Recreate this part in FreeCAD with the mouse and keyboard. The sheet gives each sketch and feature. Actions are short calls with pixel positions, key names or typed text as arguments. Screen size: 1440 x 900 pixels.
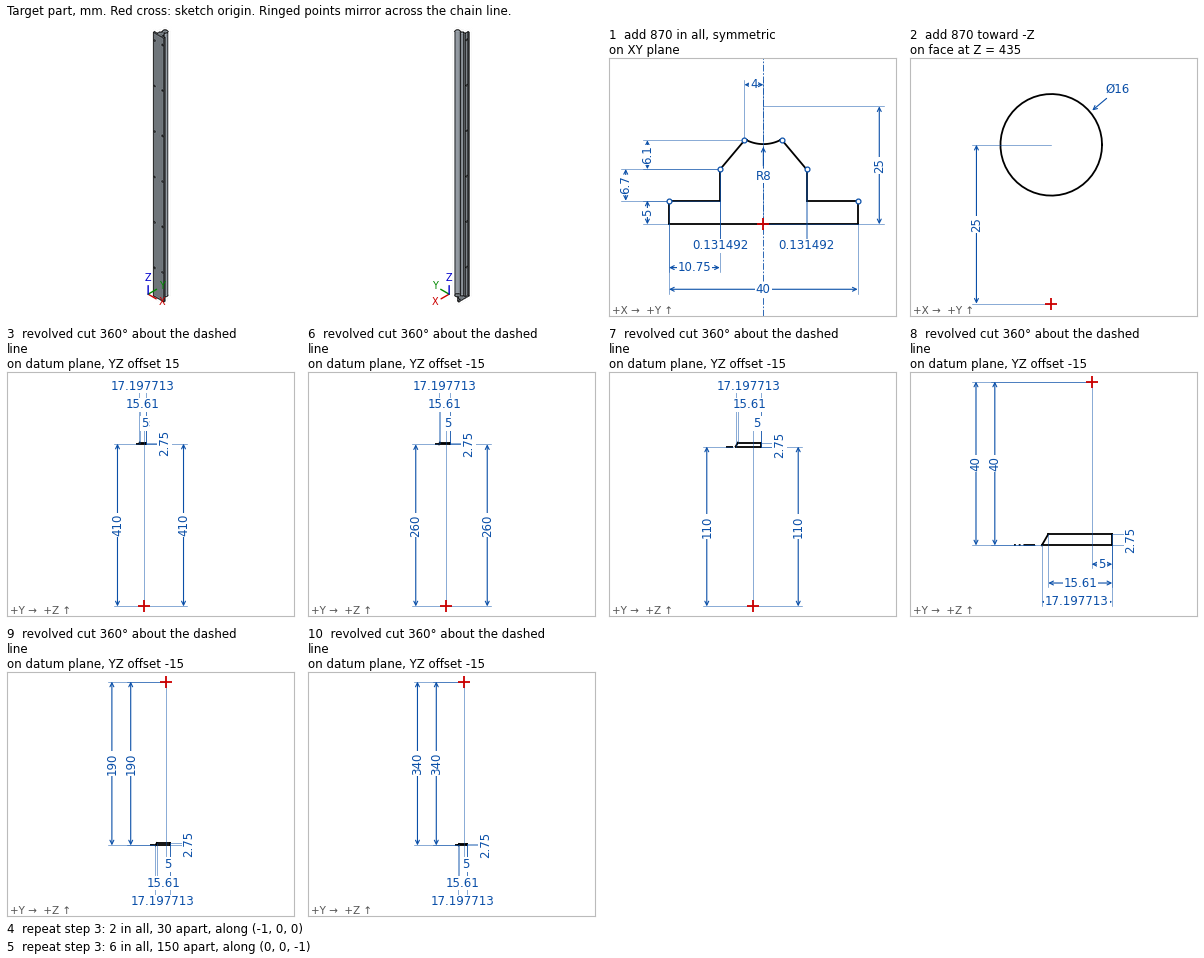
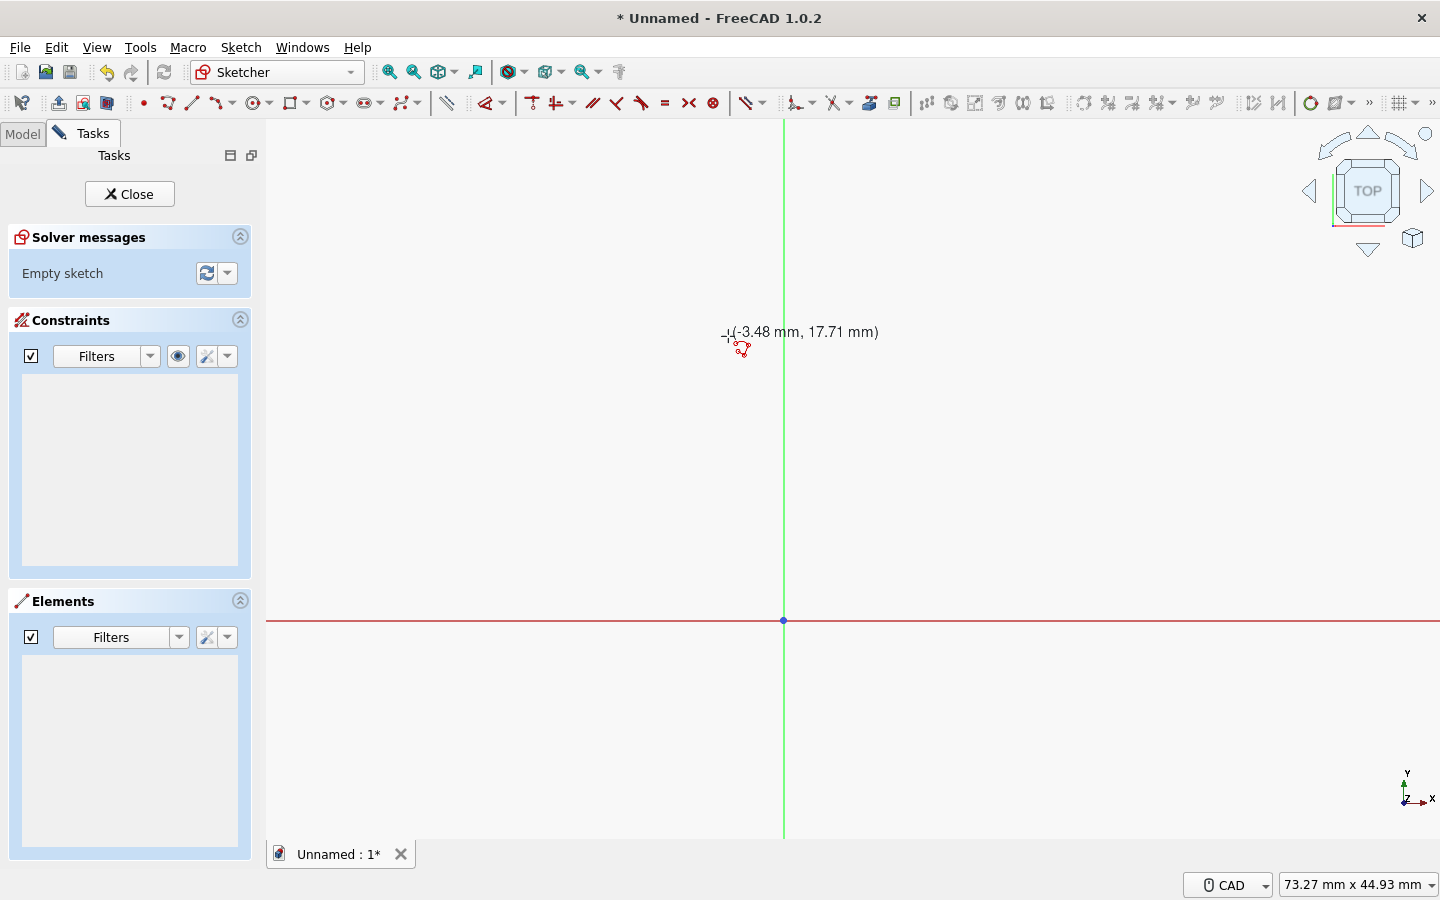
scroll(720, 336, up, 4)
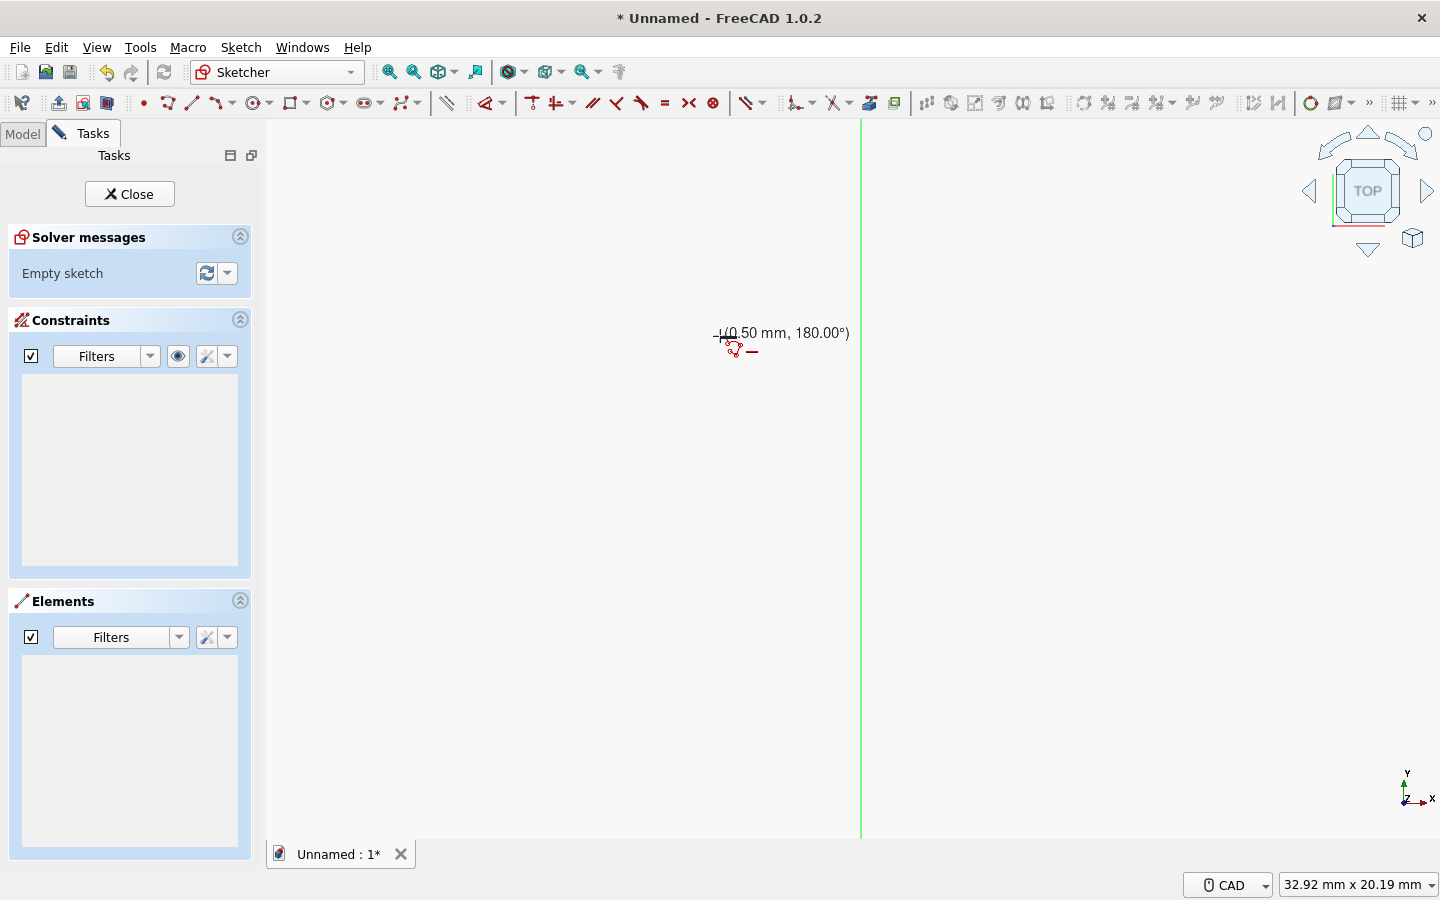
click(719, 336)
click(536, 552)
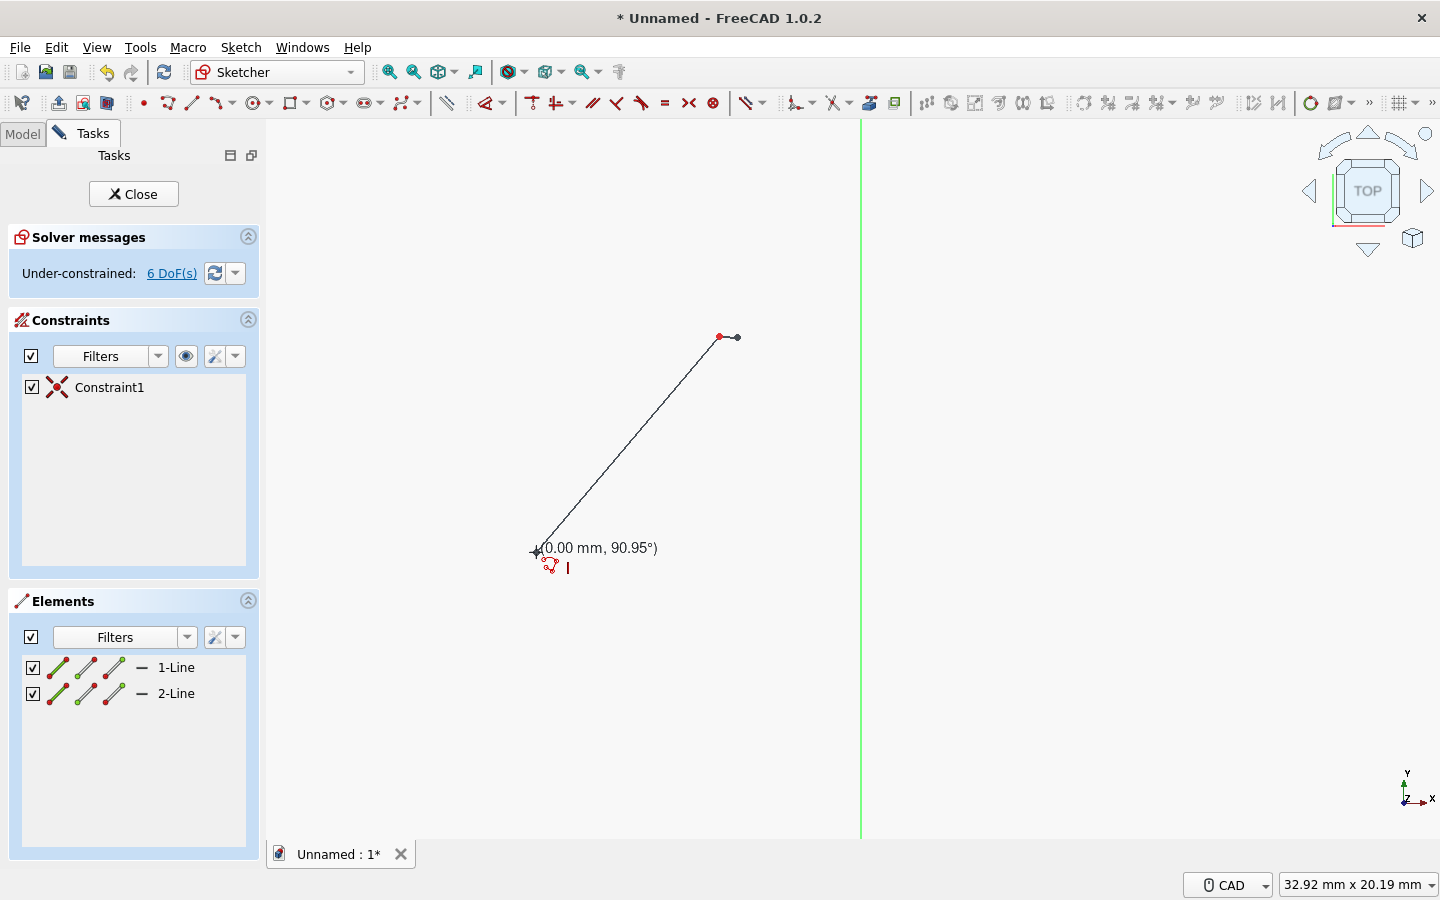
scroll(531, 552, up, 7)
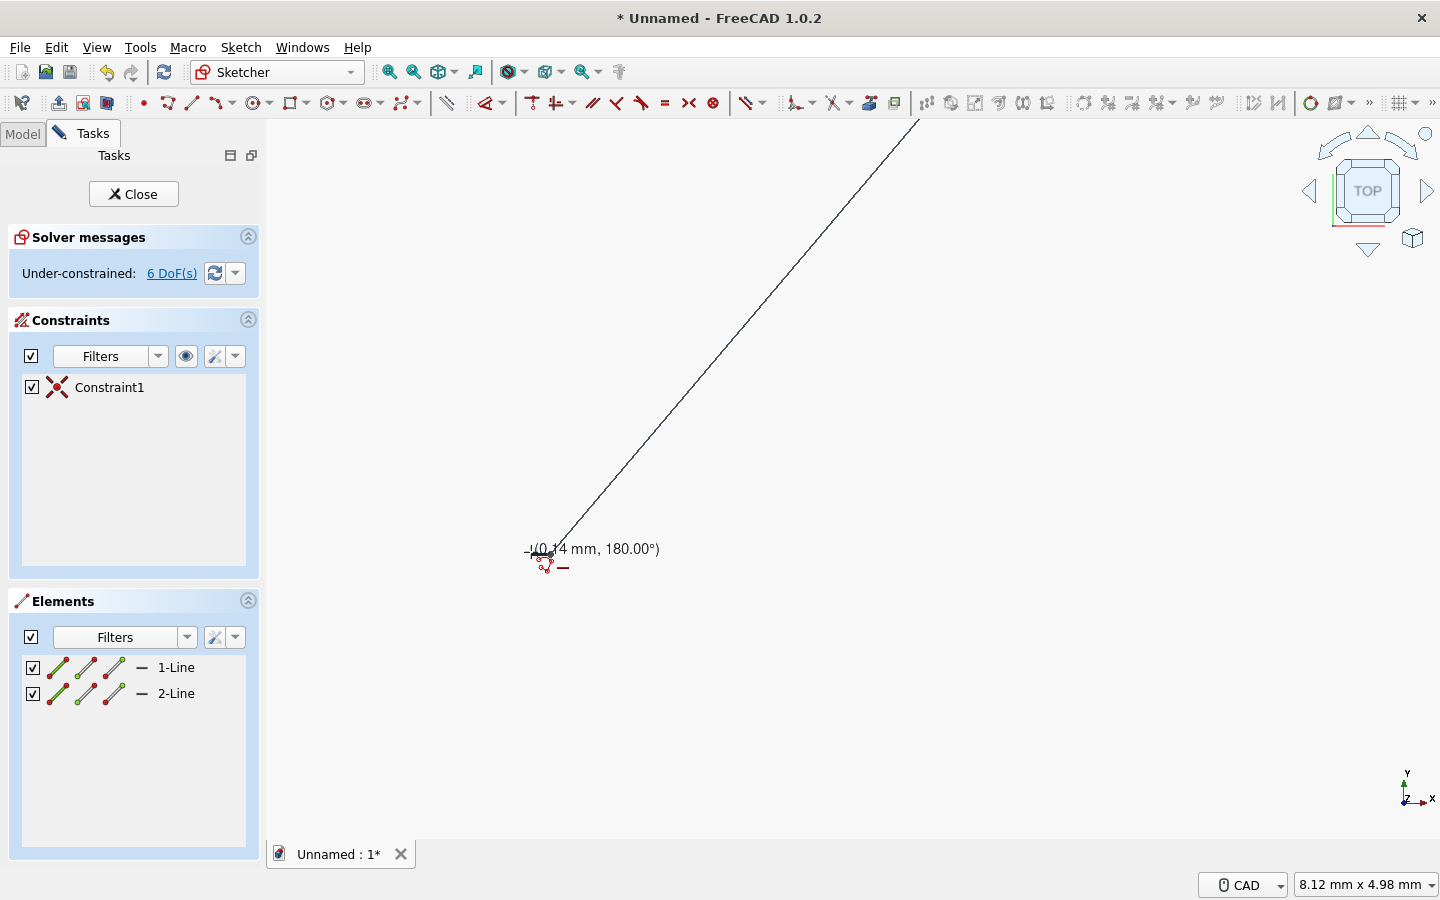
click(532, 550)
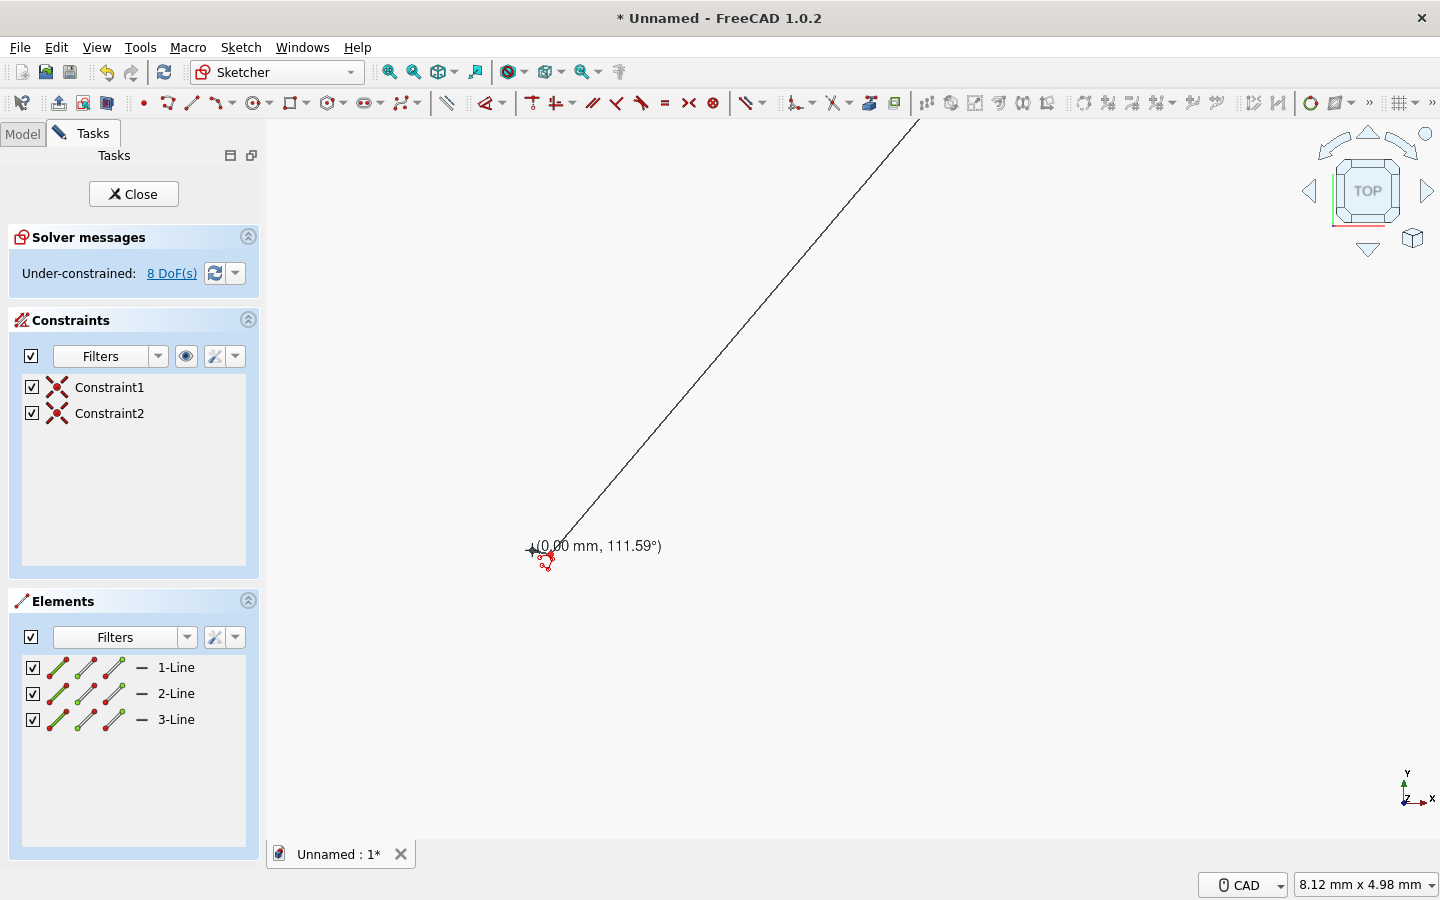
scroll(649, 420, down, 11)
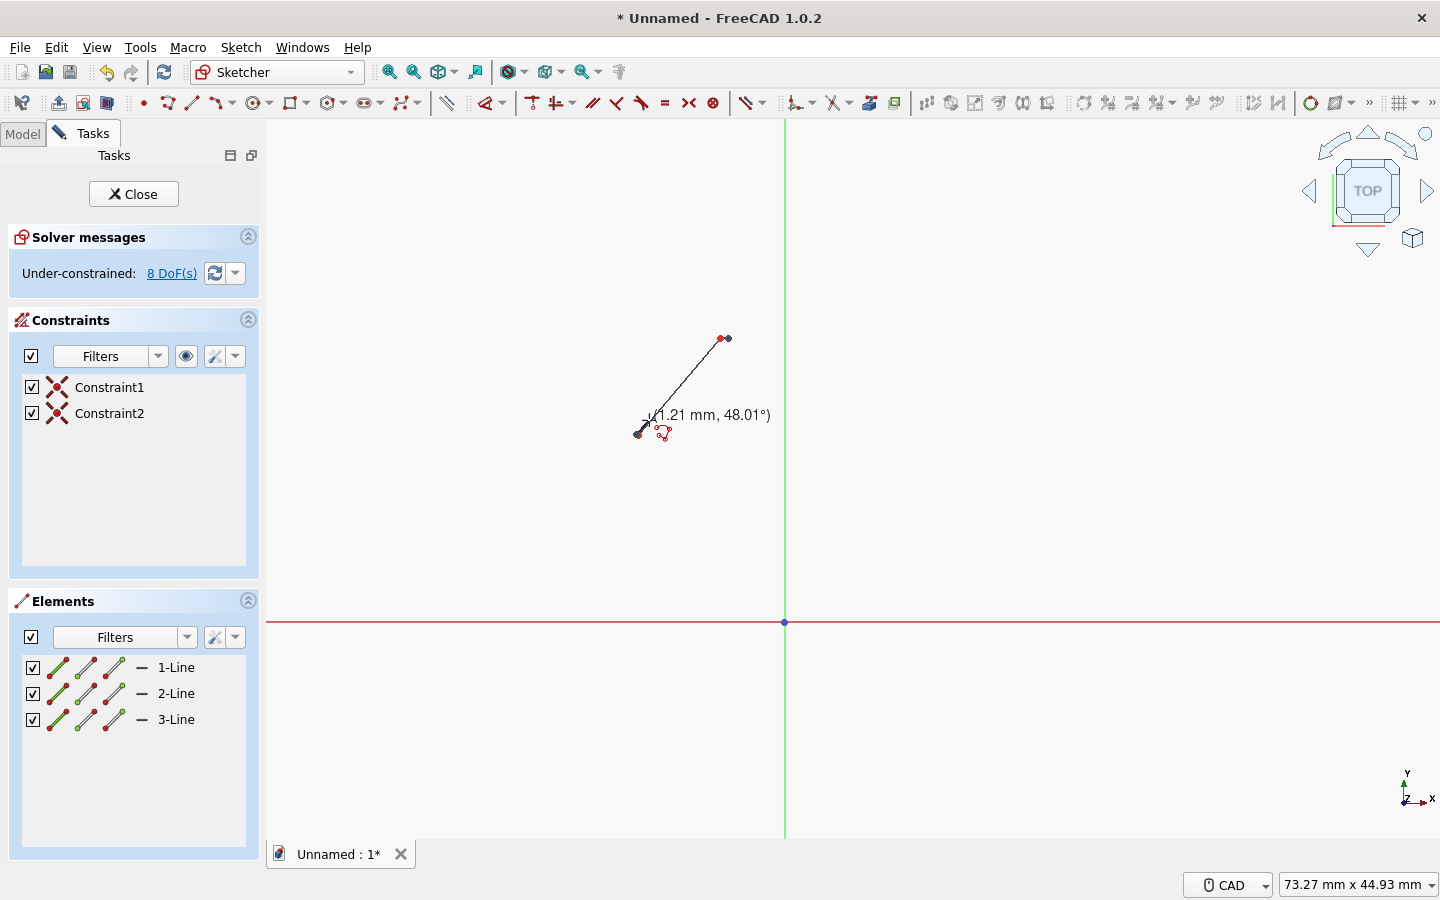
click(636, 542)
click(464, 542)
click(464, 622)
click(1105, 613)
click(1105, 542)
click(933, 542)
click(933, 435)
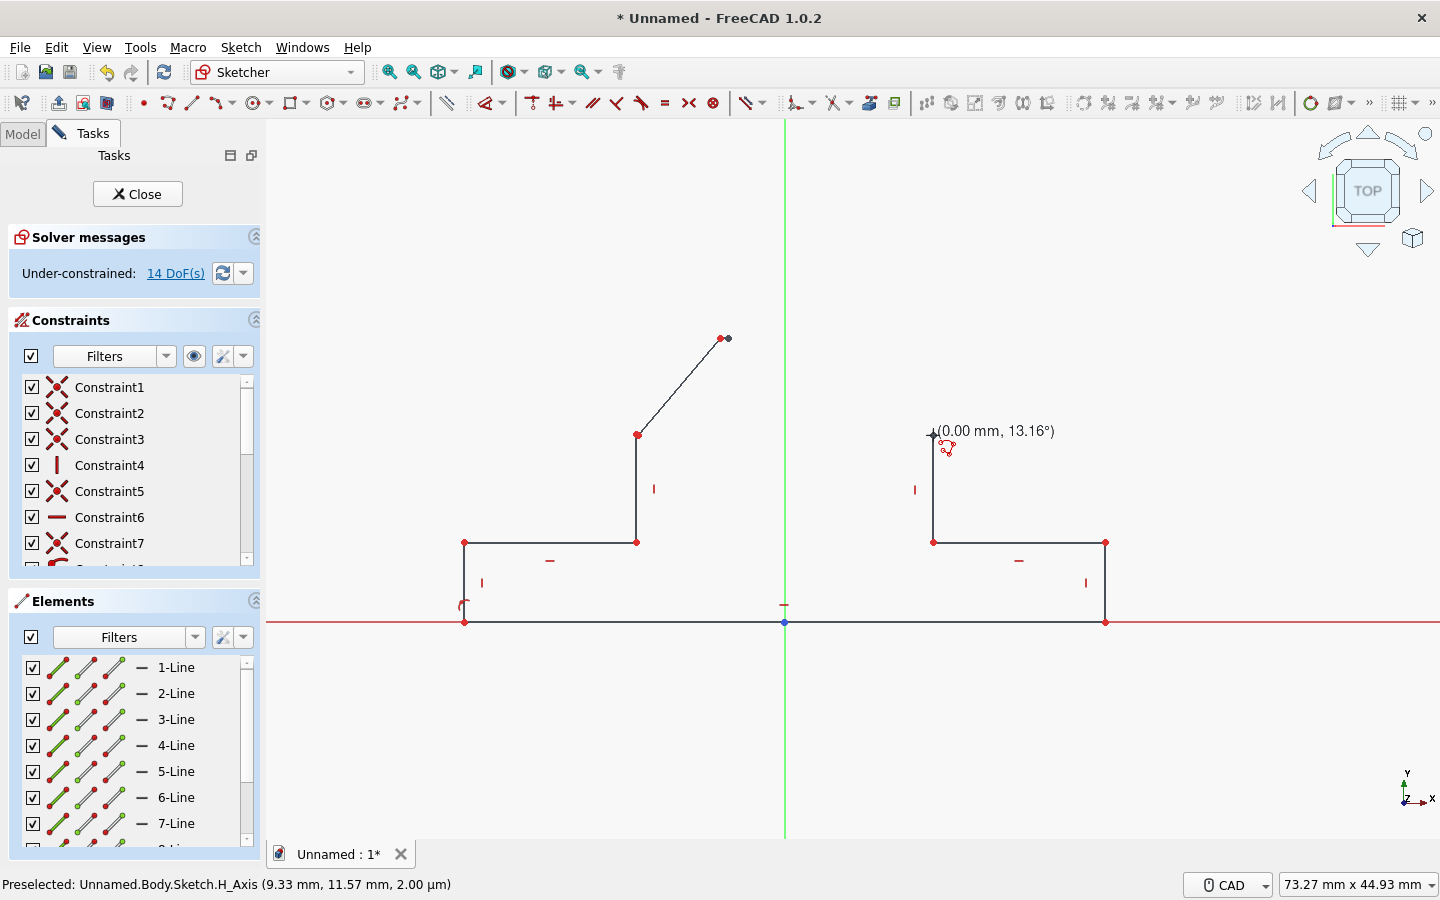
scroll(931, 435, up, 11)